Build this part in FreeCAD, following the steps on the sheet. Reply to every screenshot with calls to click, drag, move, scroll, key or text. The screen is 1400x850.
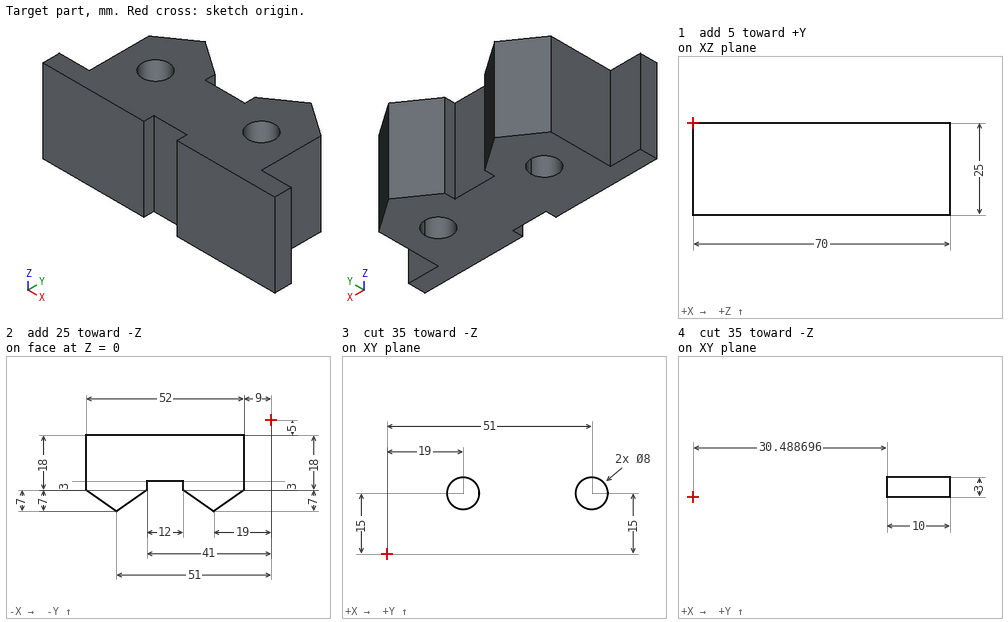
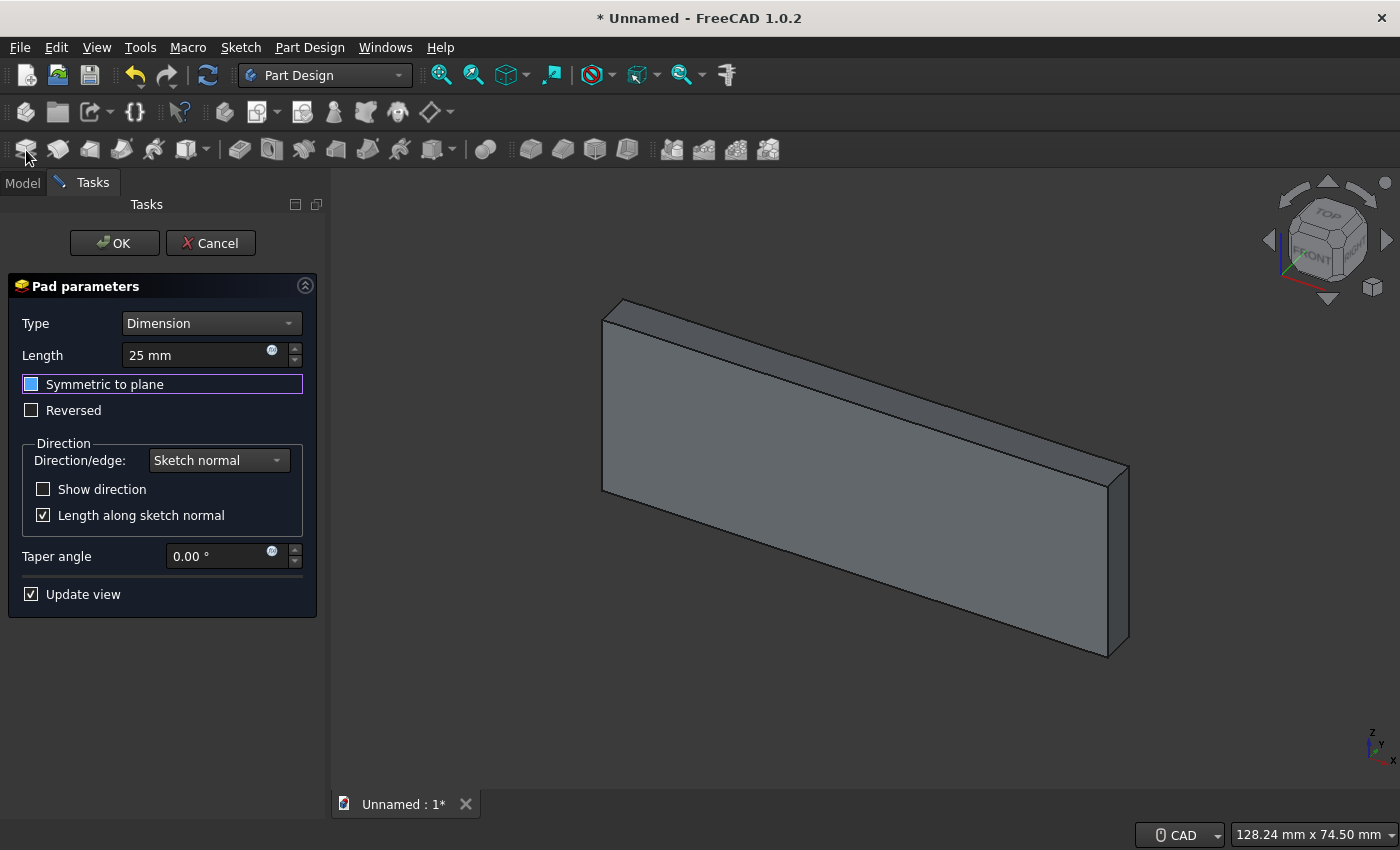
click(30, 410)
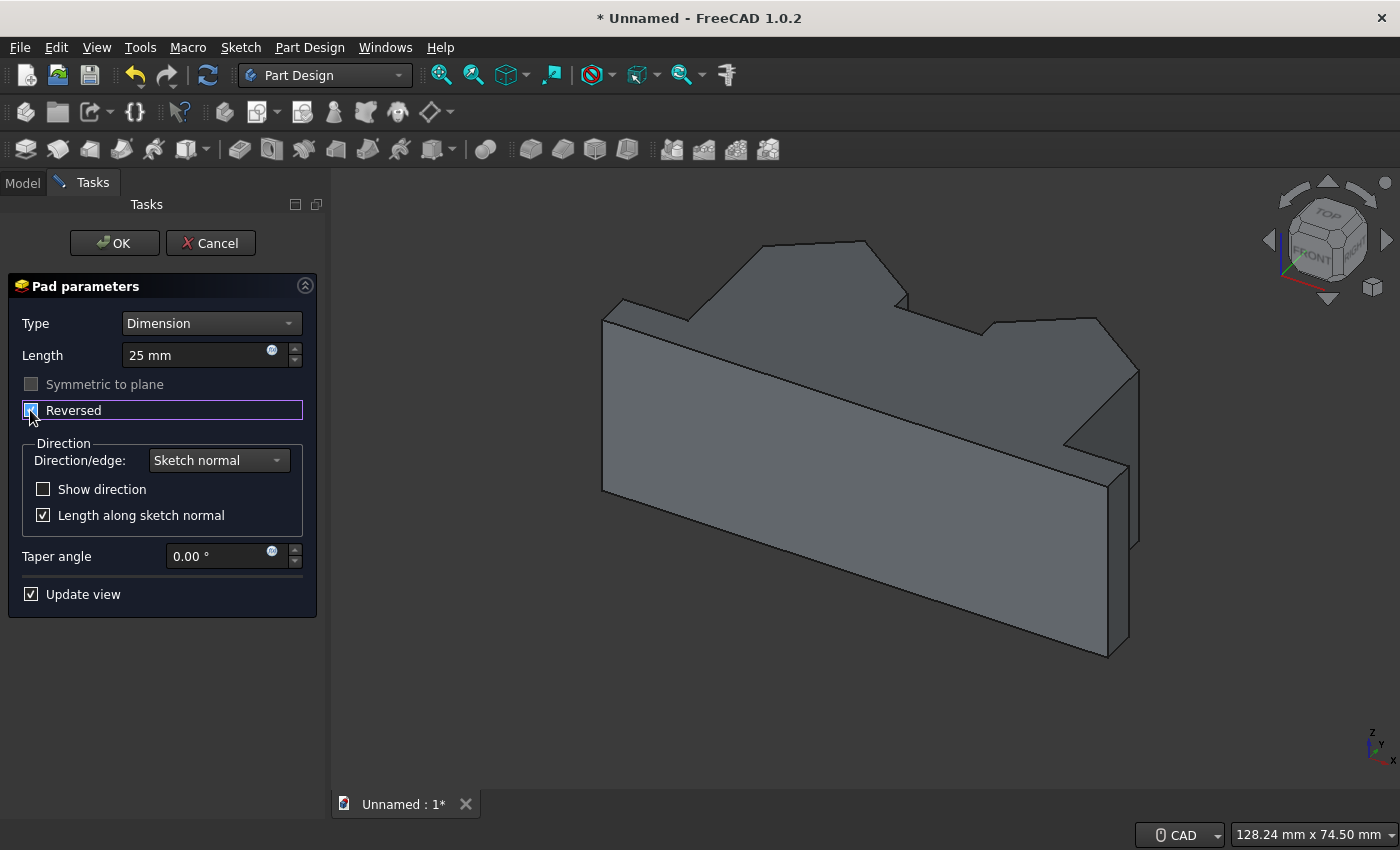
click(115, 243)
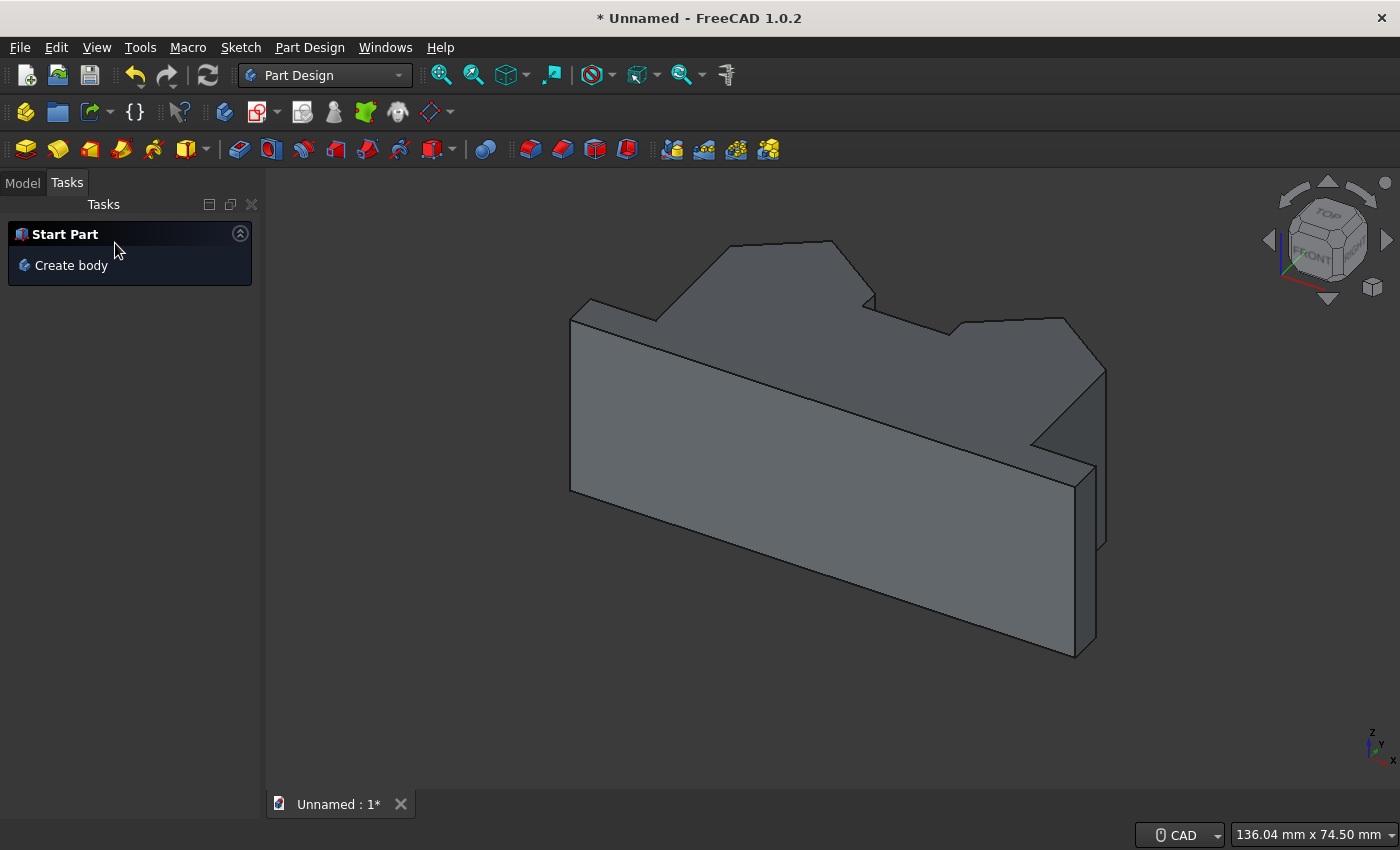
click(258, 112)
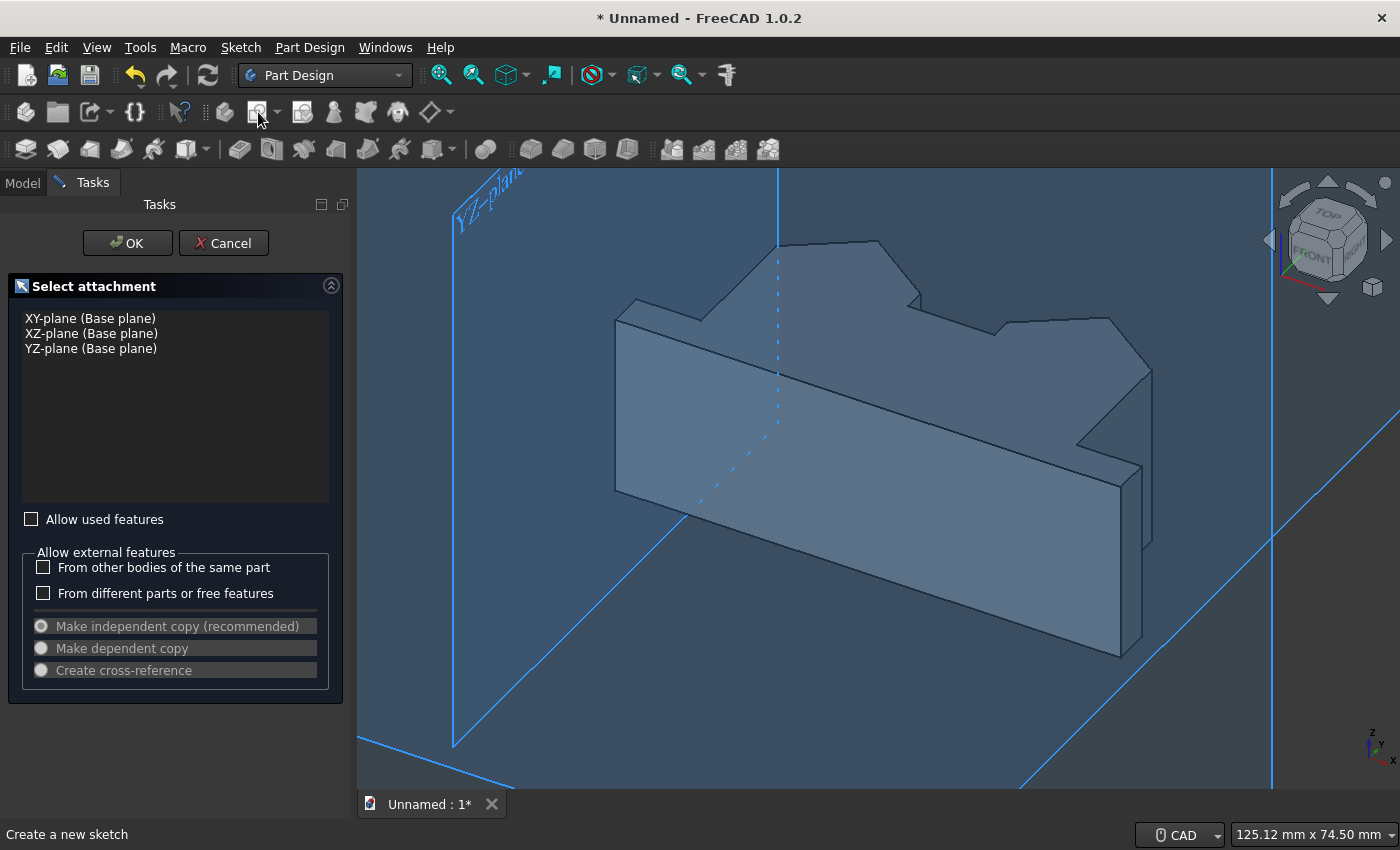
click(82, 318)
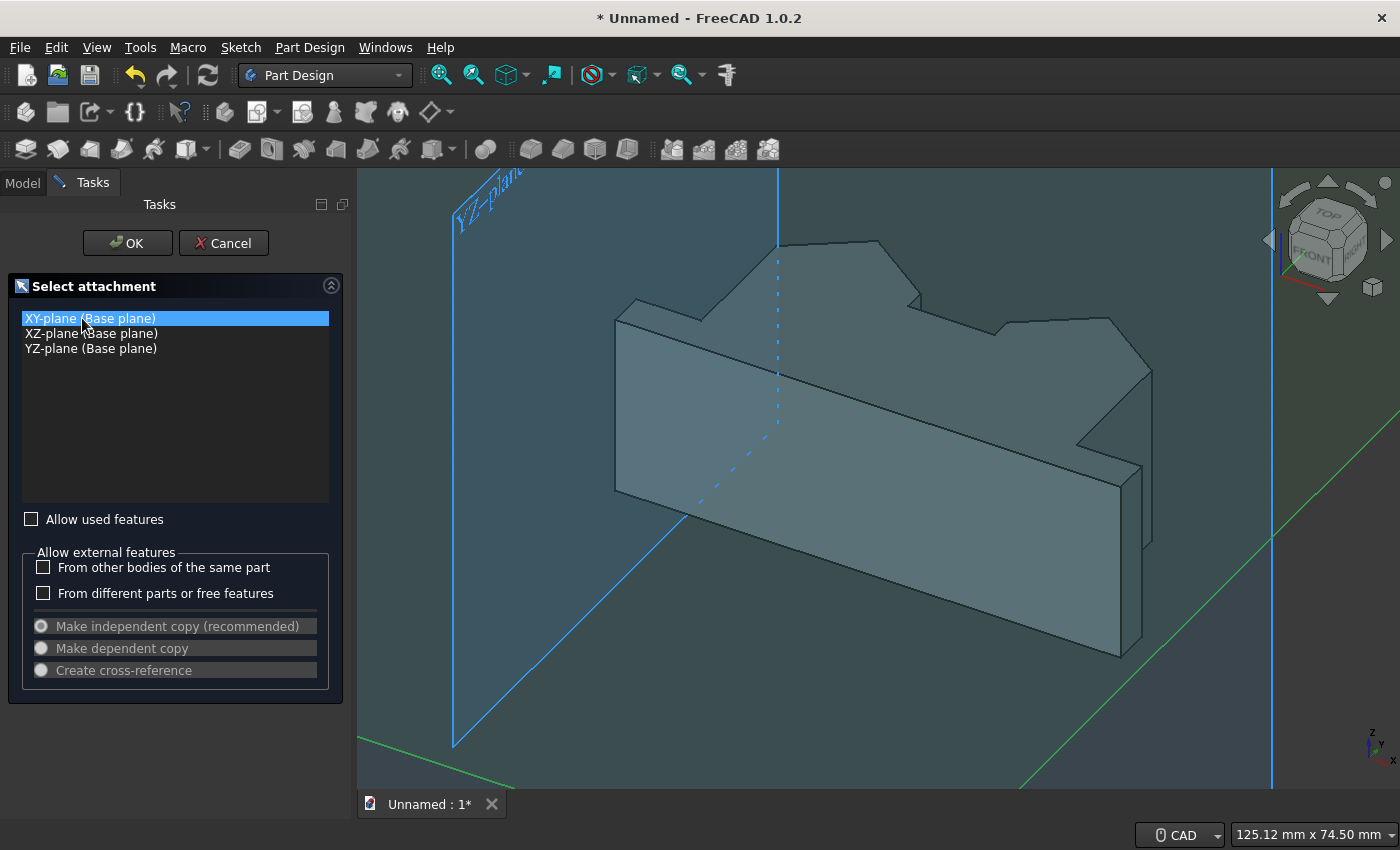
click(128, 243)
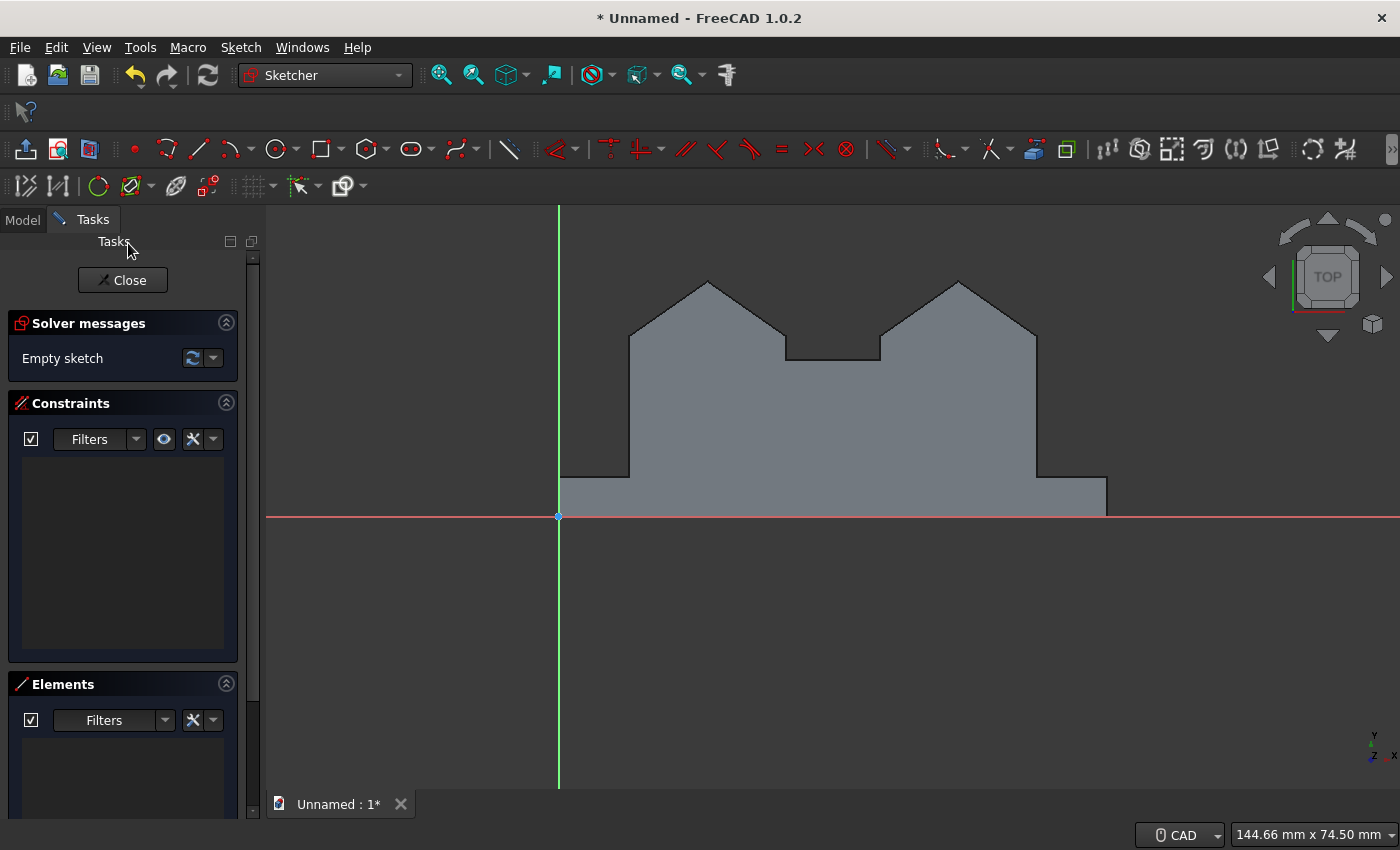
scroll(794, 331, up, 2)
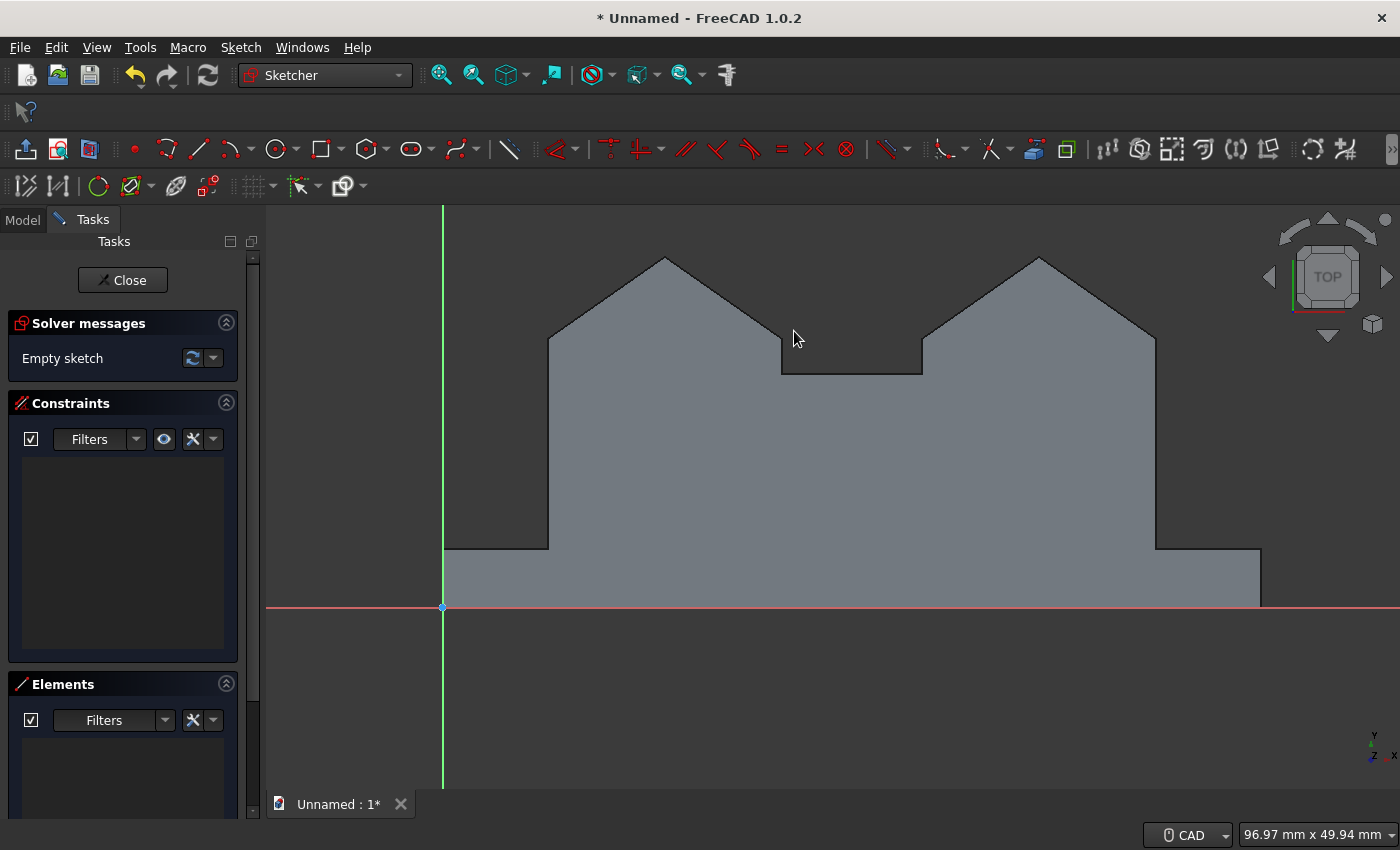
key(g)
key(c)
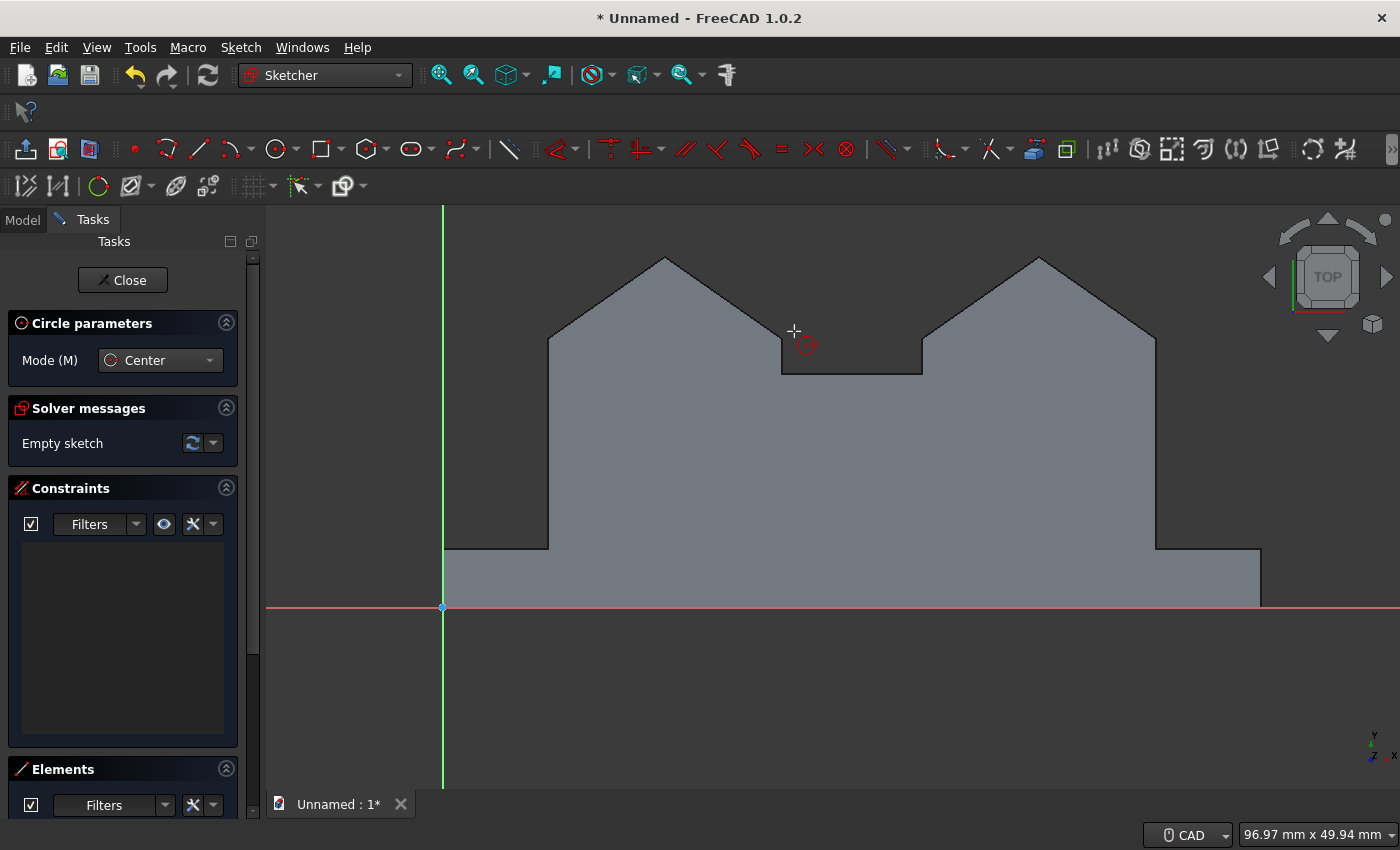
click(1039, 432)
move(1072, 399)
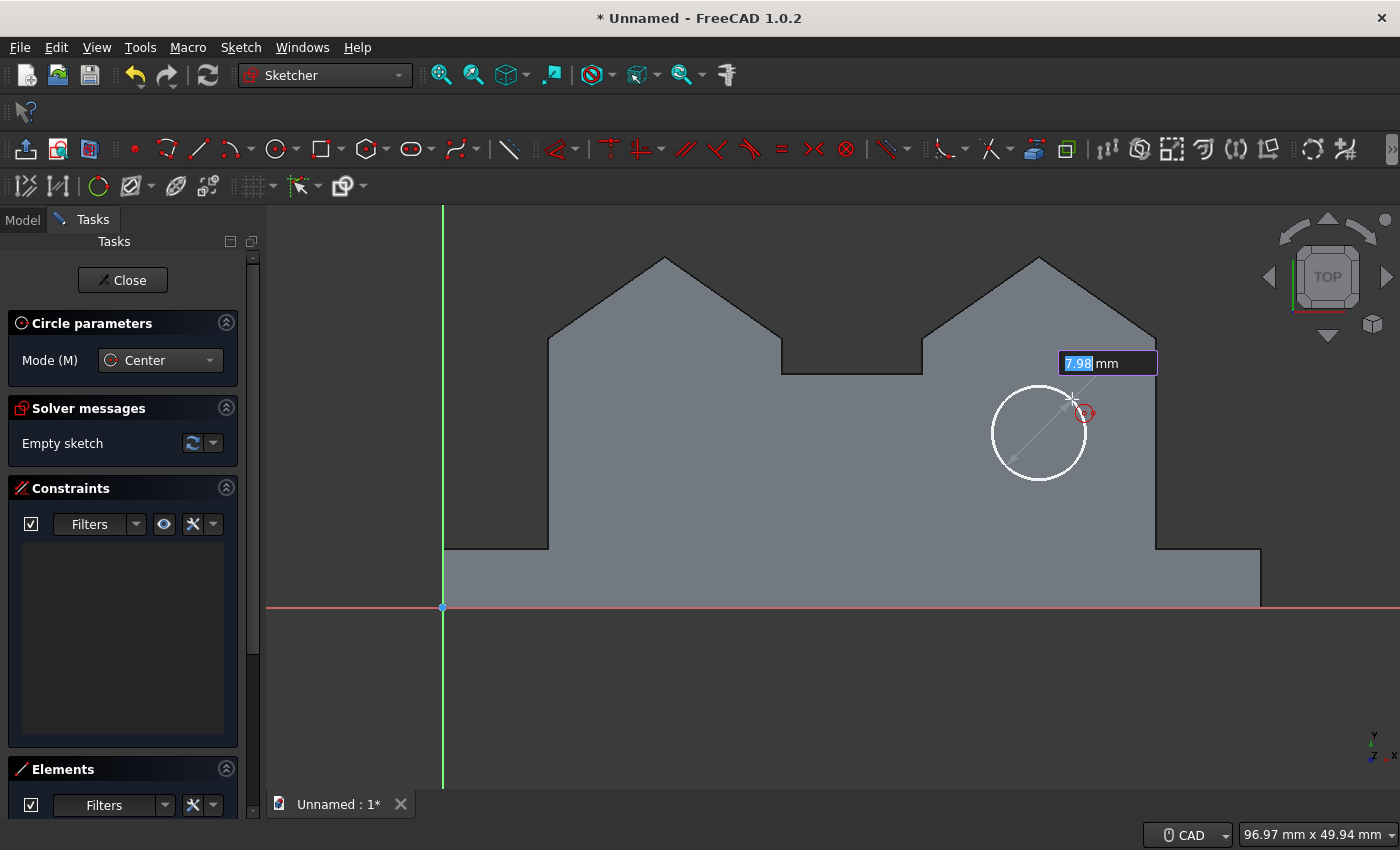
text(8)
key(Return)